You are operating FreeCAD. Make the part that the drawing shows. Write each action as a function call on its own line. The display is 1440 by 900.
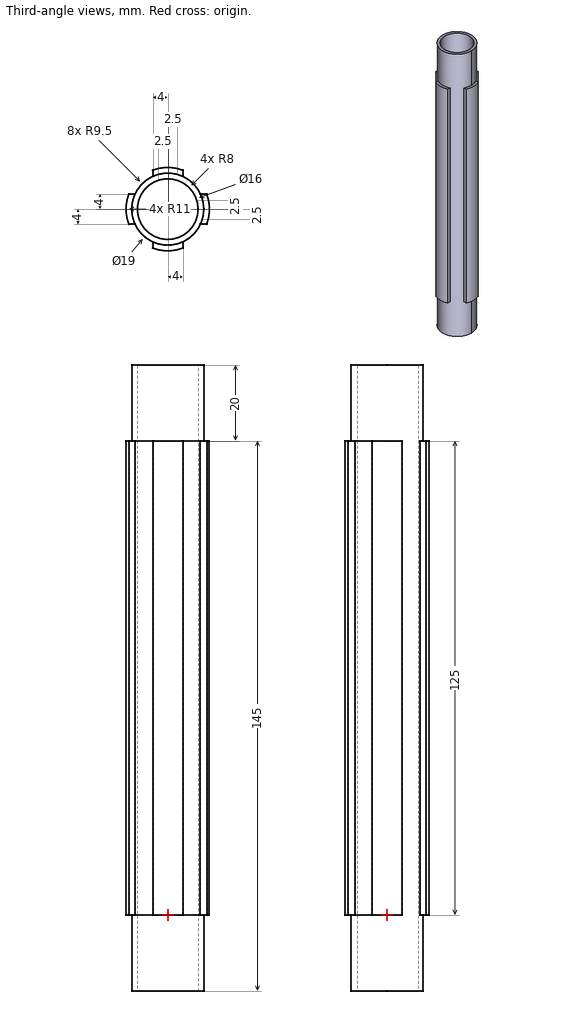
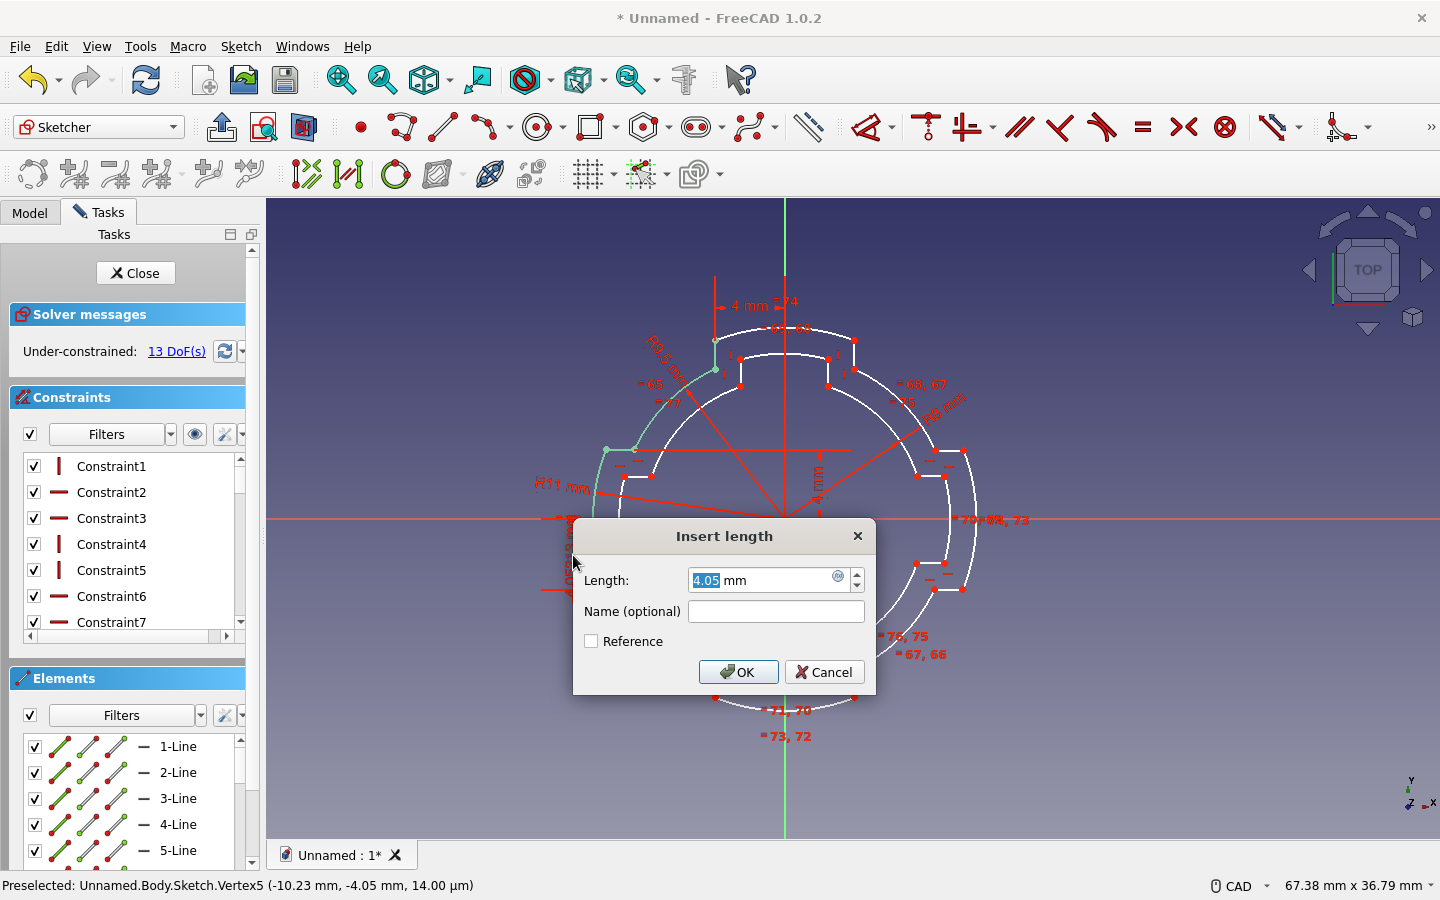
text(4)
key(Return)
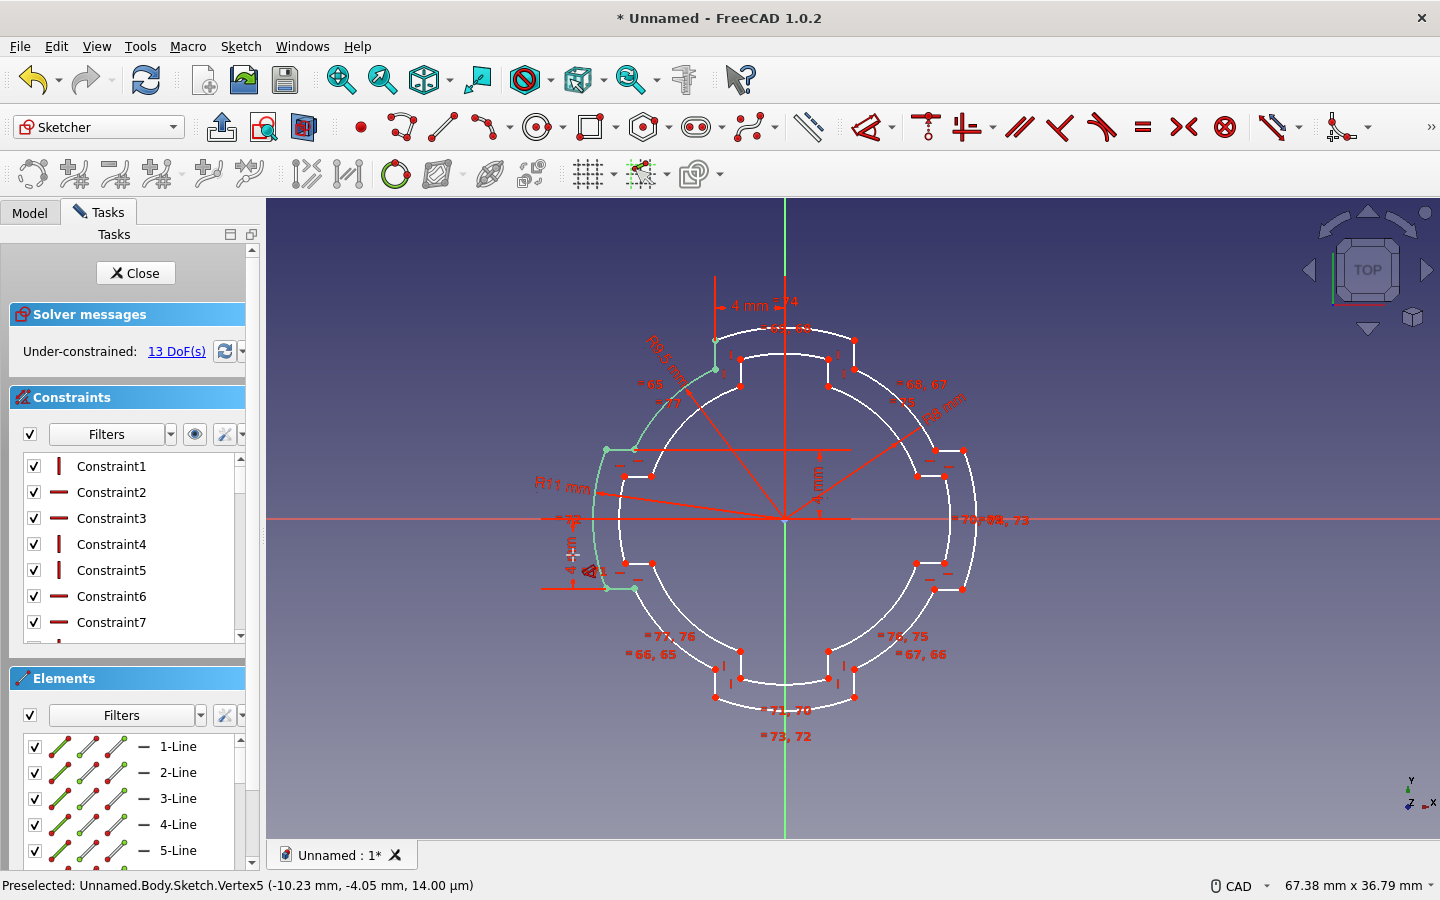
click(715, 669)
click(734, 485)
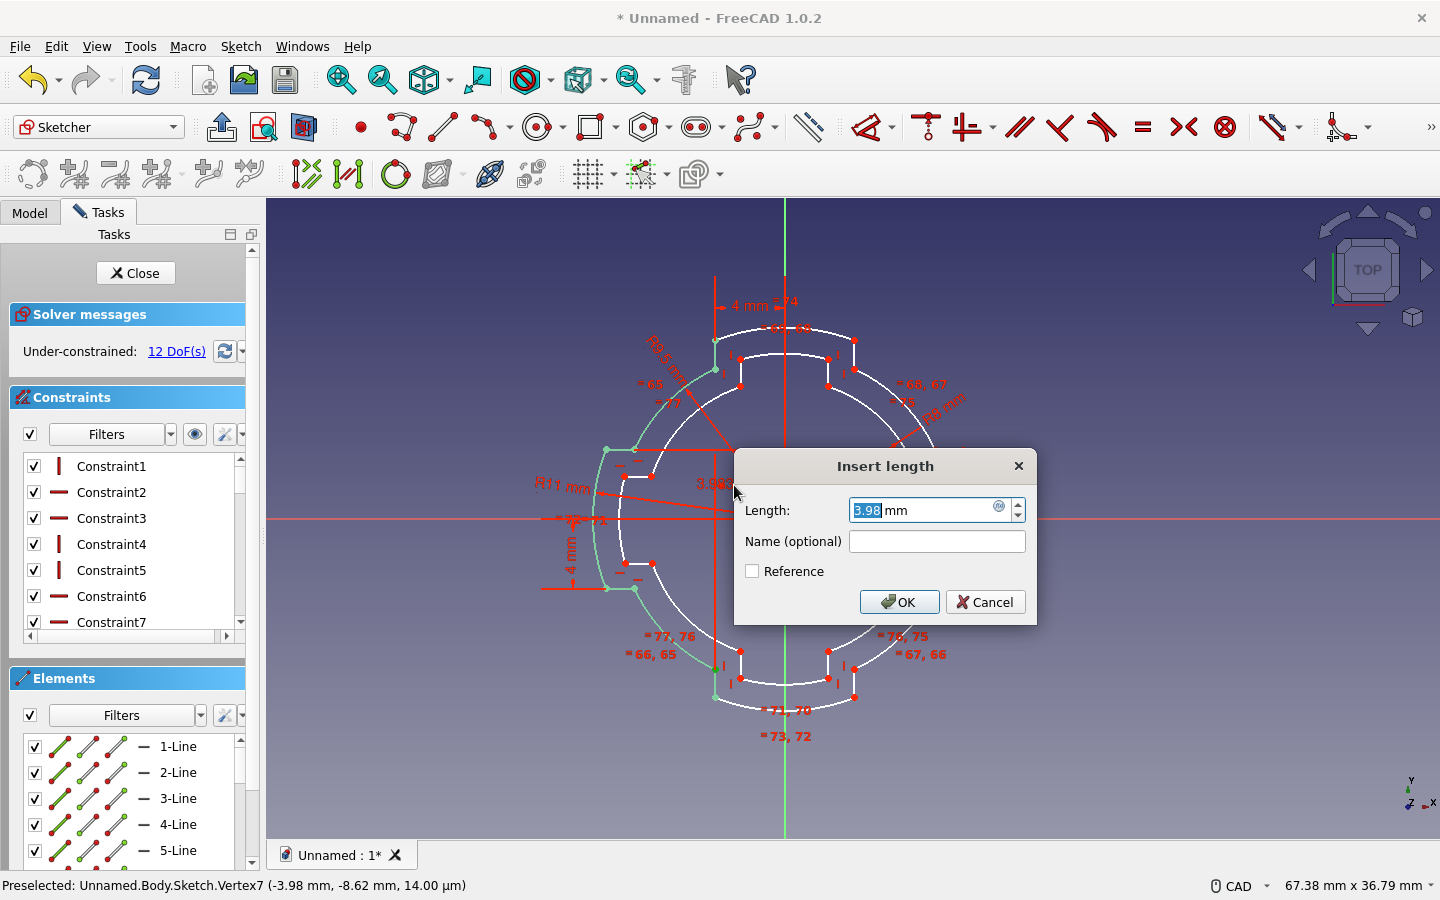
text(4)
key(Return)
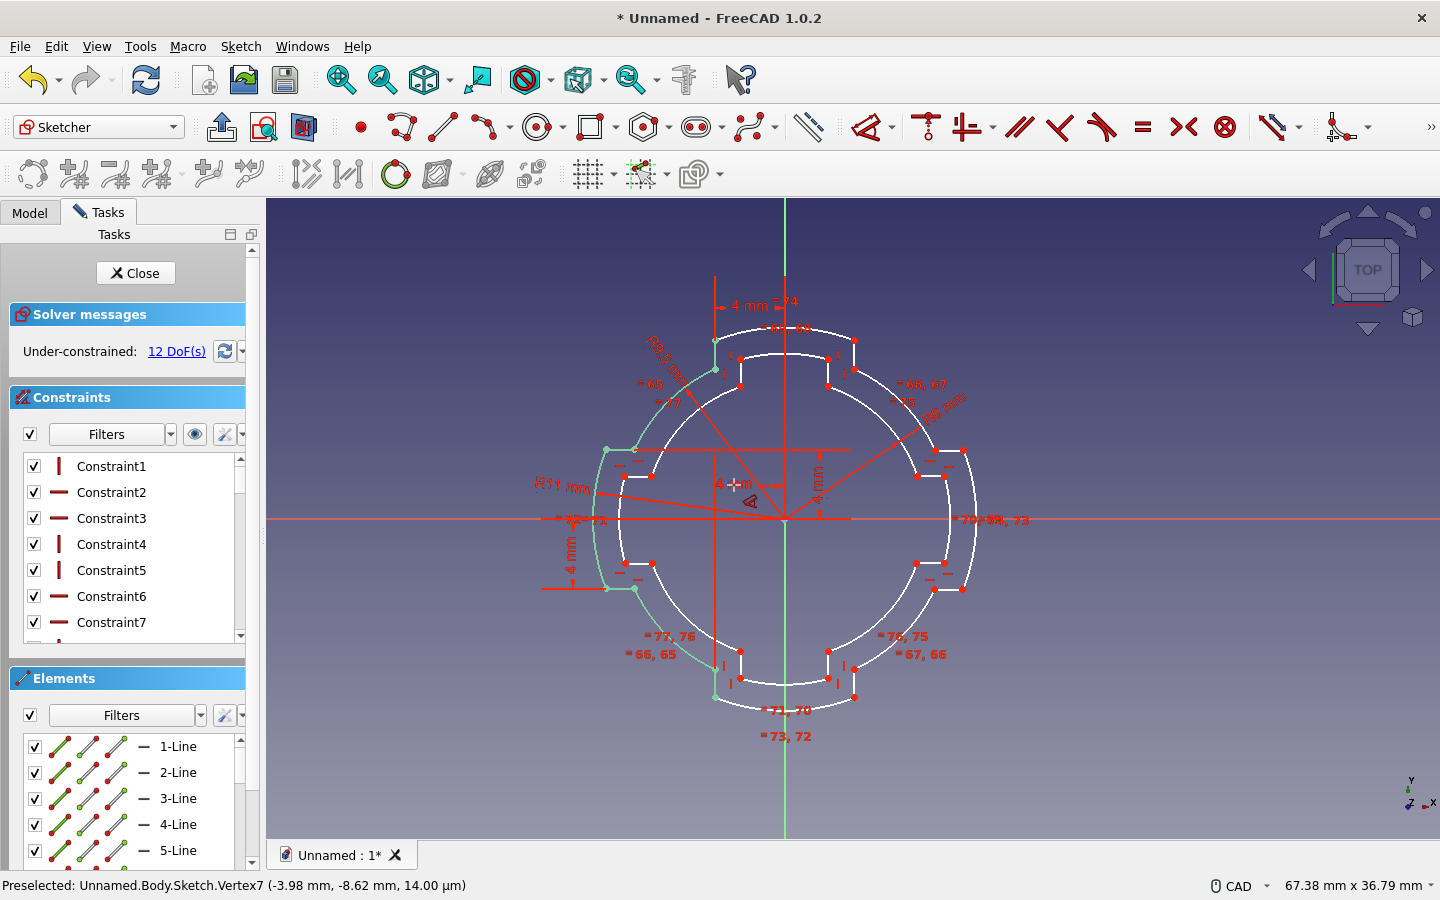
click(854, 698)
click(820, 732)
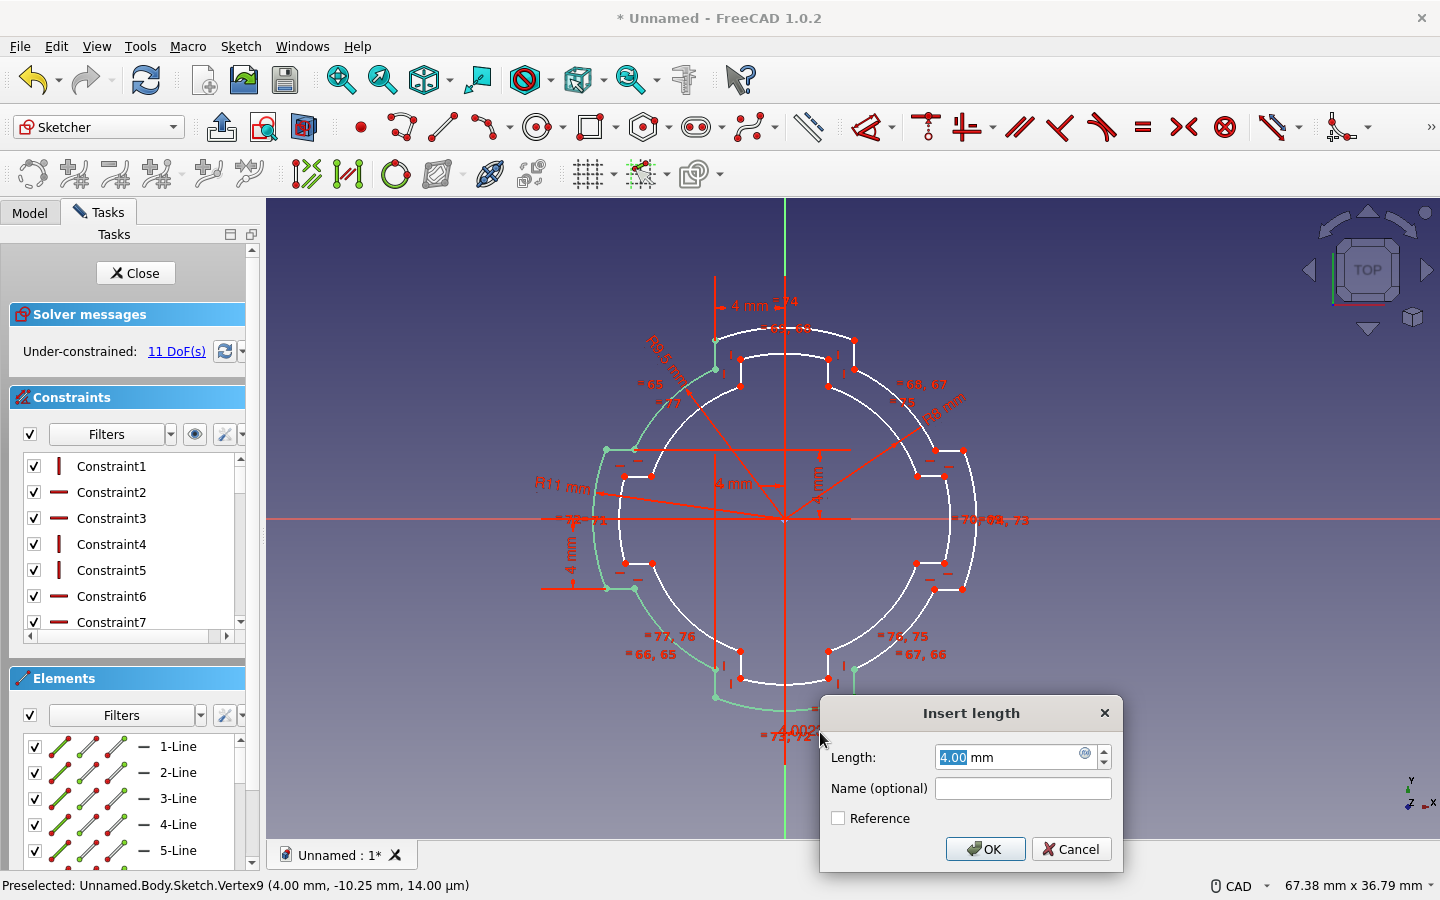
text(4)
key(Return)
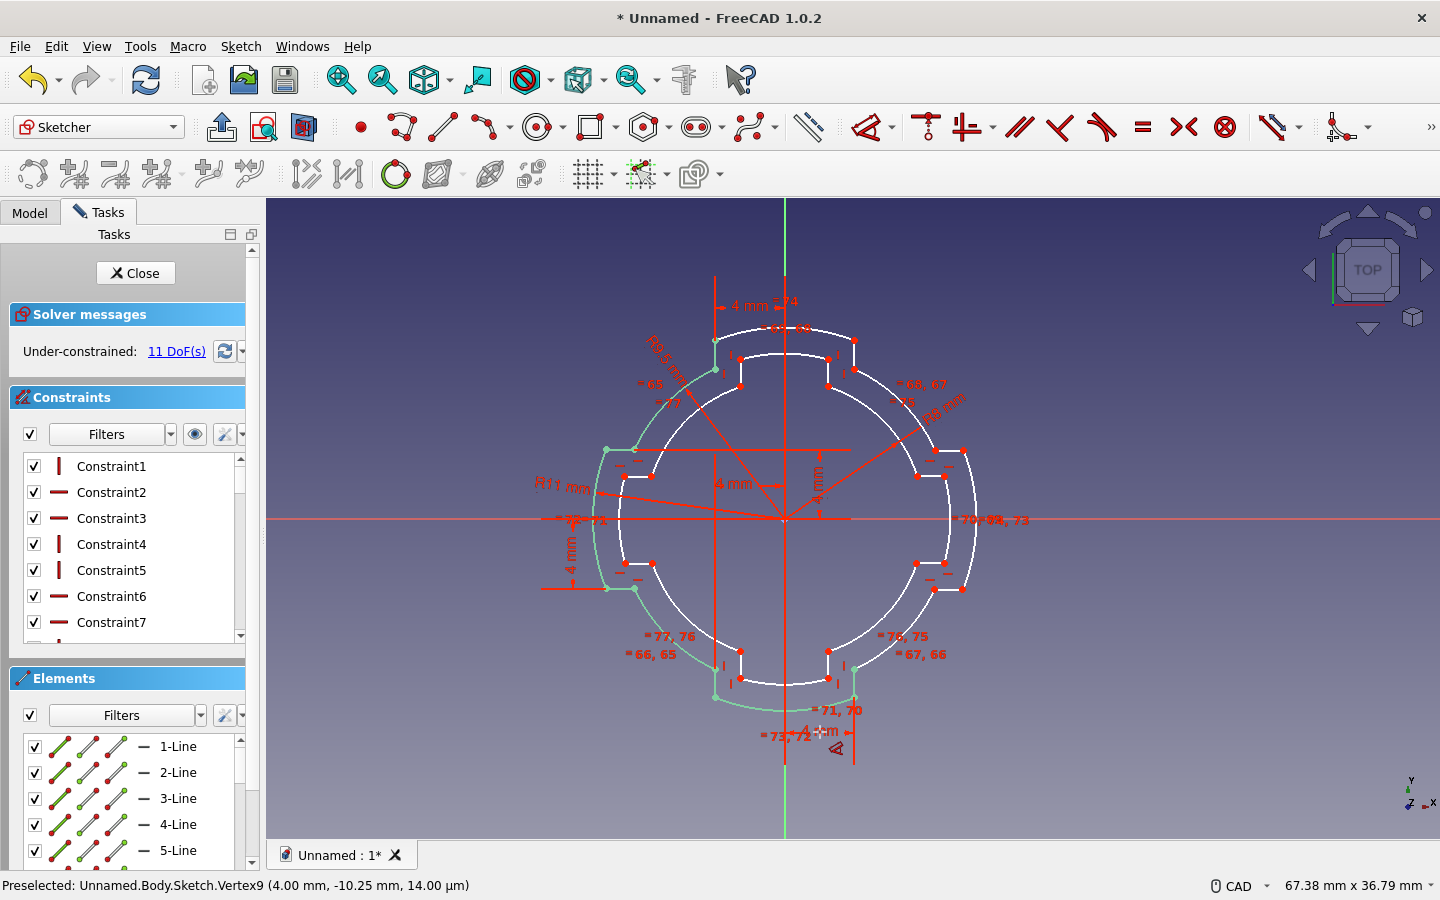
click(934, 590)
click(751, 555)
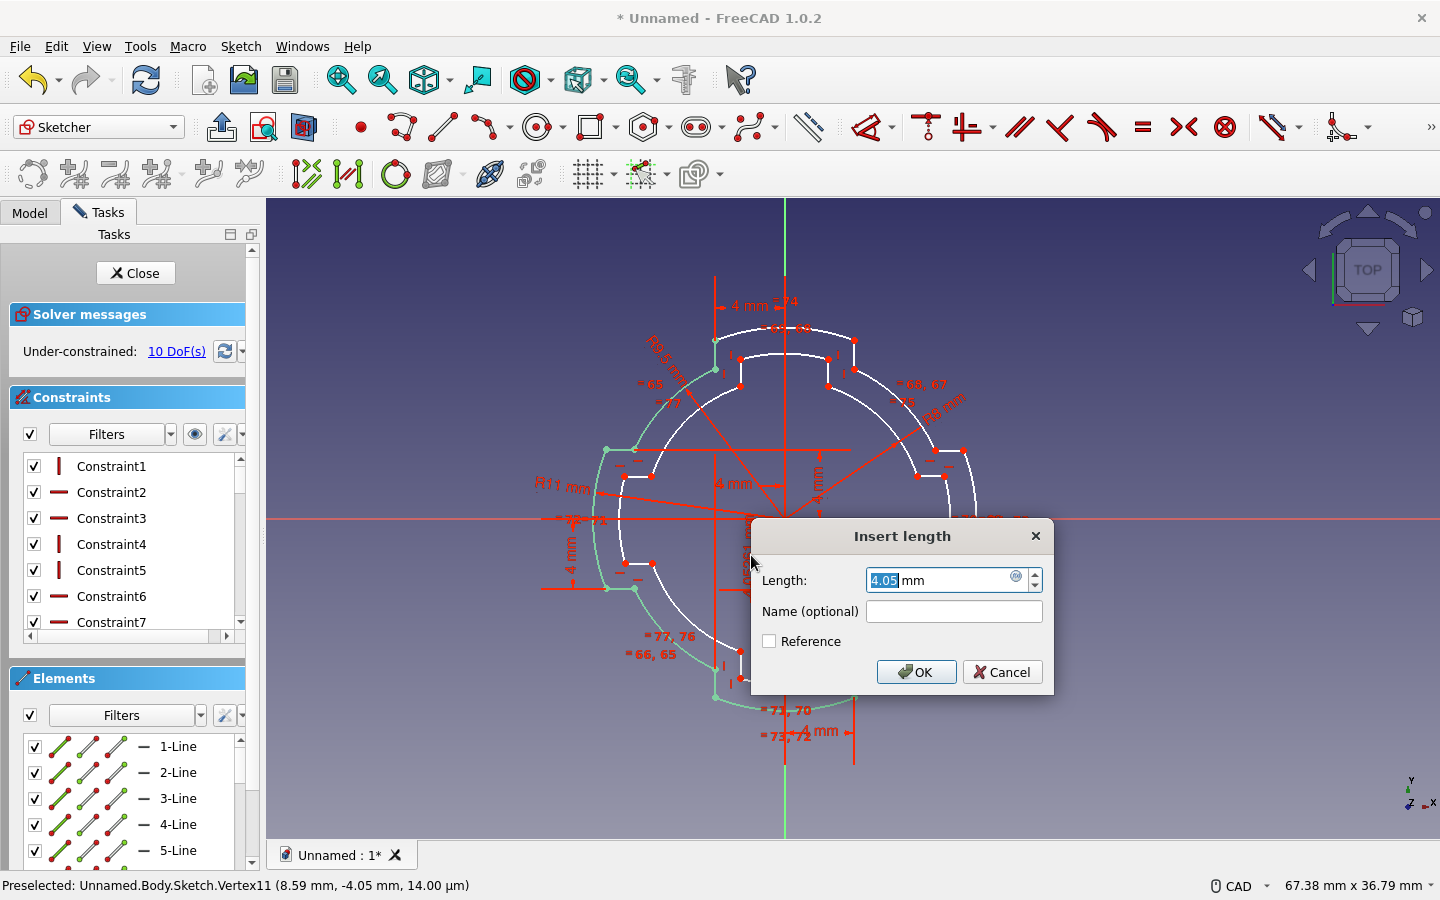
text(4)
key(Return)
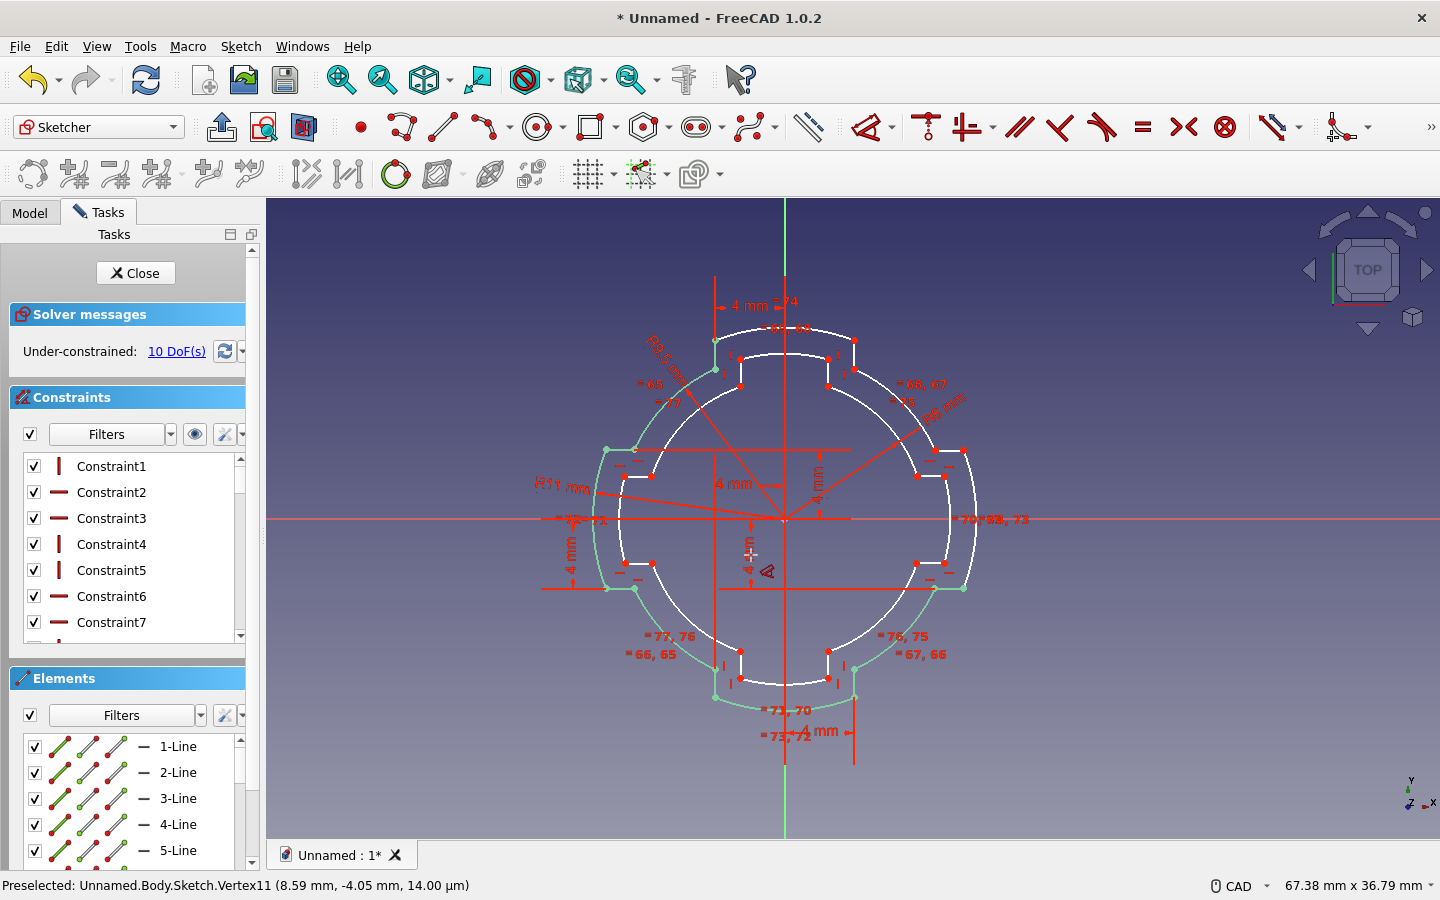
click(964, 451)
click(998, 485)